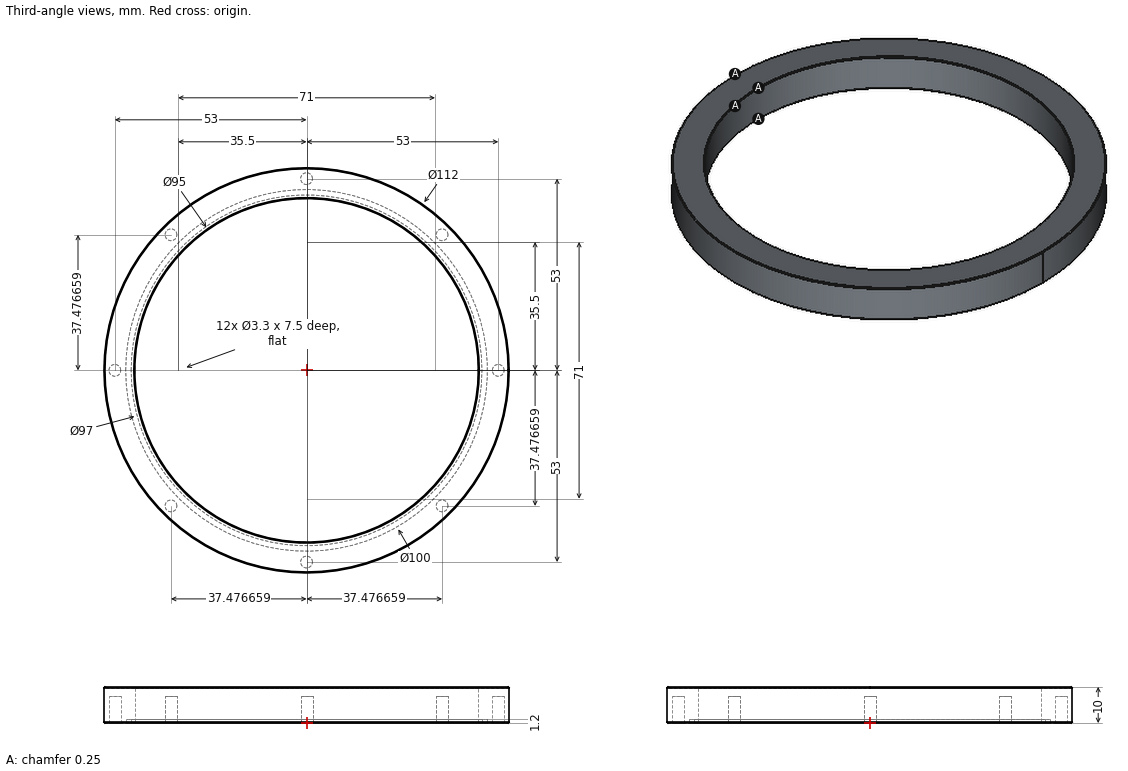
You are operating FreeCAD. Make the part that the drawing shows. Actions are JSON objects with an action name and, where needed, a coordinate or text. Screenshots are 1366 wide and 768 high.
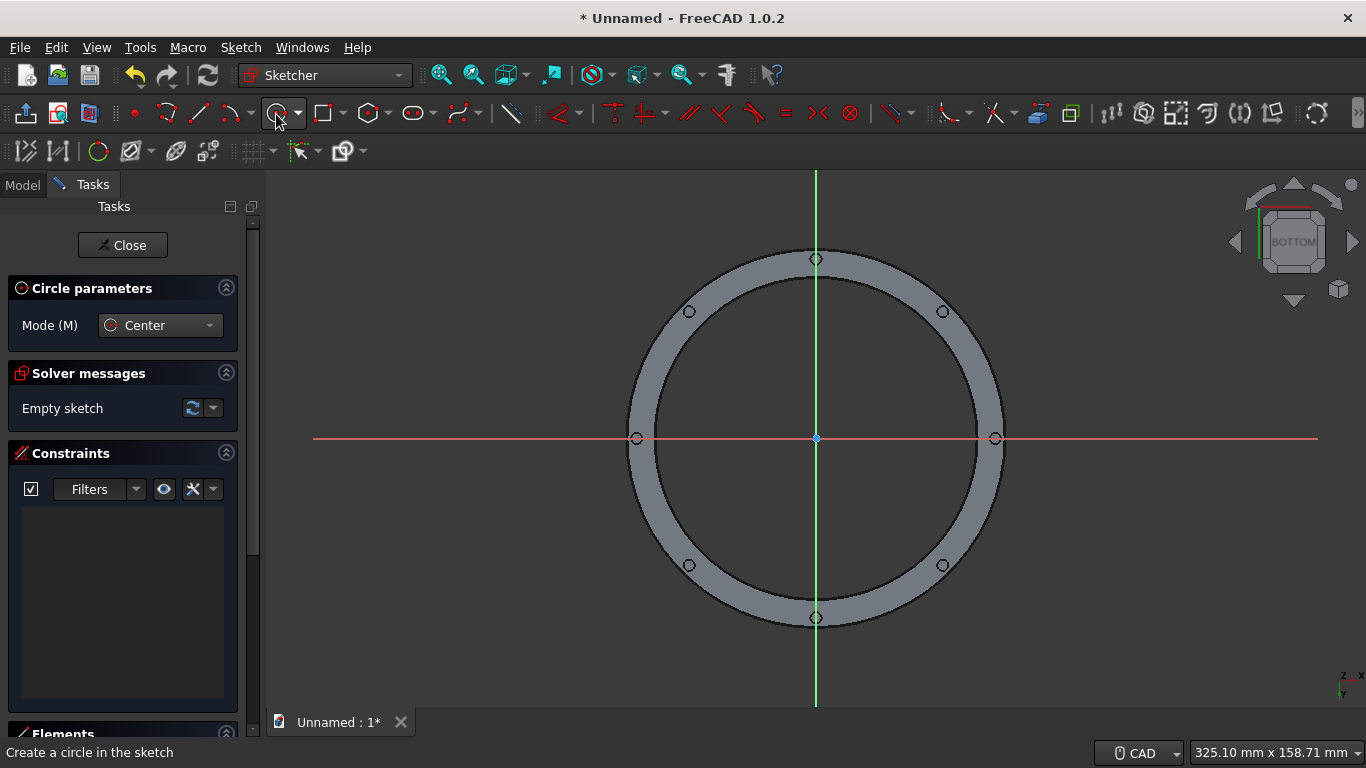
{"action": "left_click", "coordinate": [816, 438]}
{"action": "mouse_move", "coordinate": [936, 319]}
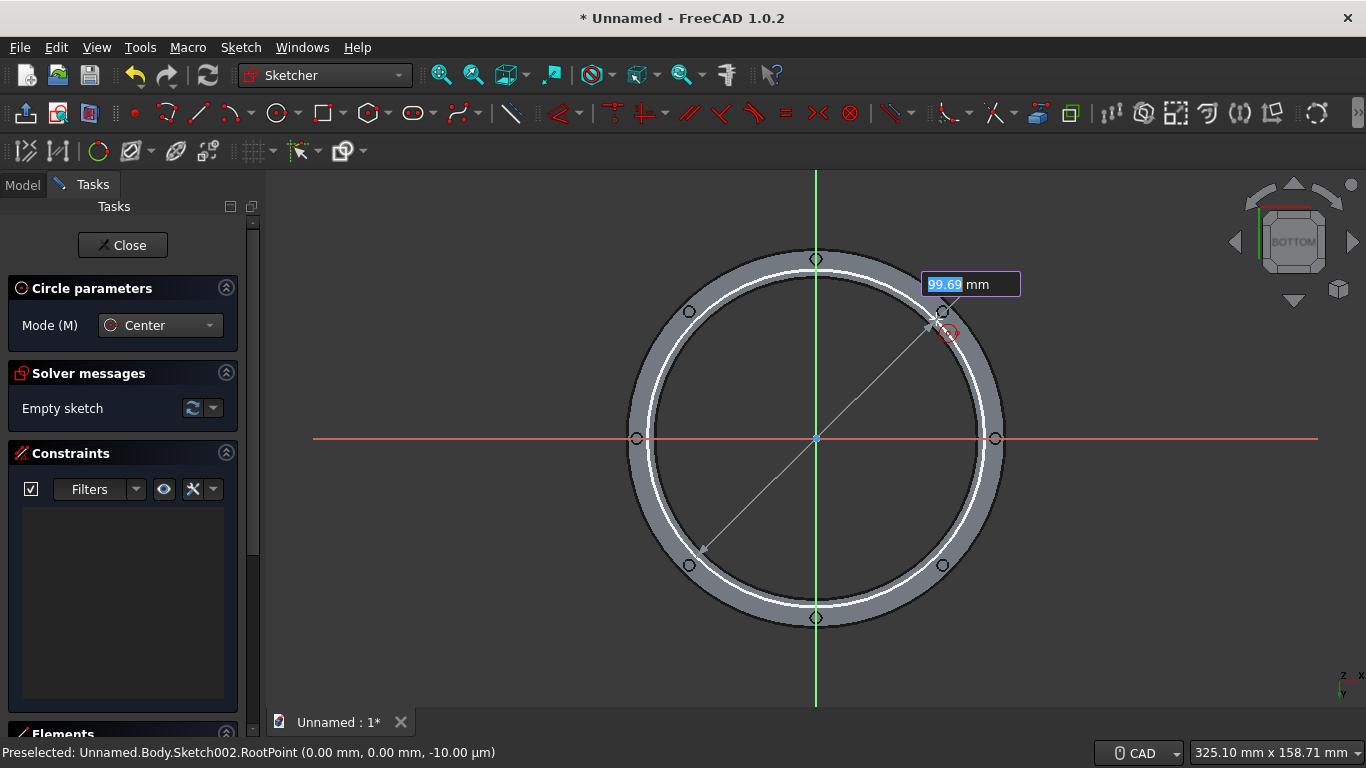
{"action": "type", "text": "100"}
{"action": "key", "text": "Return"}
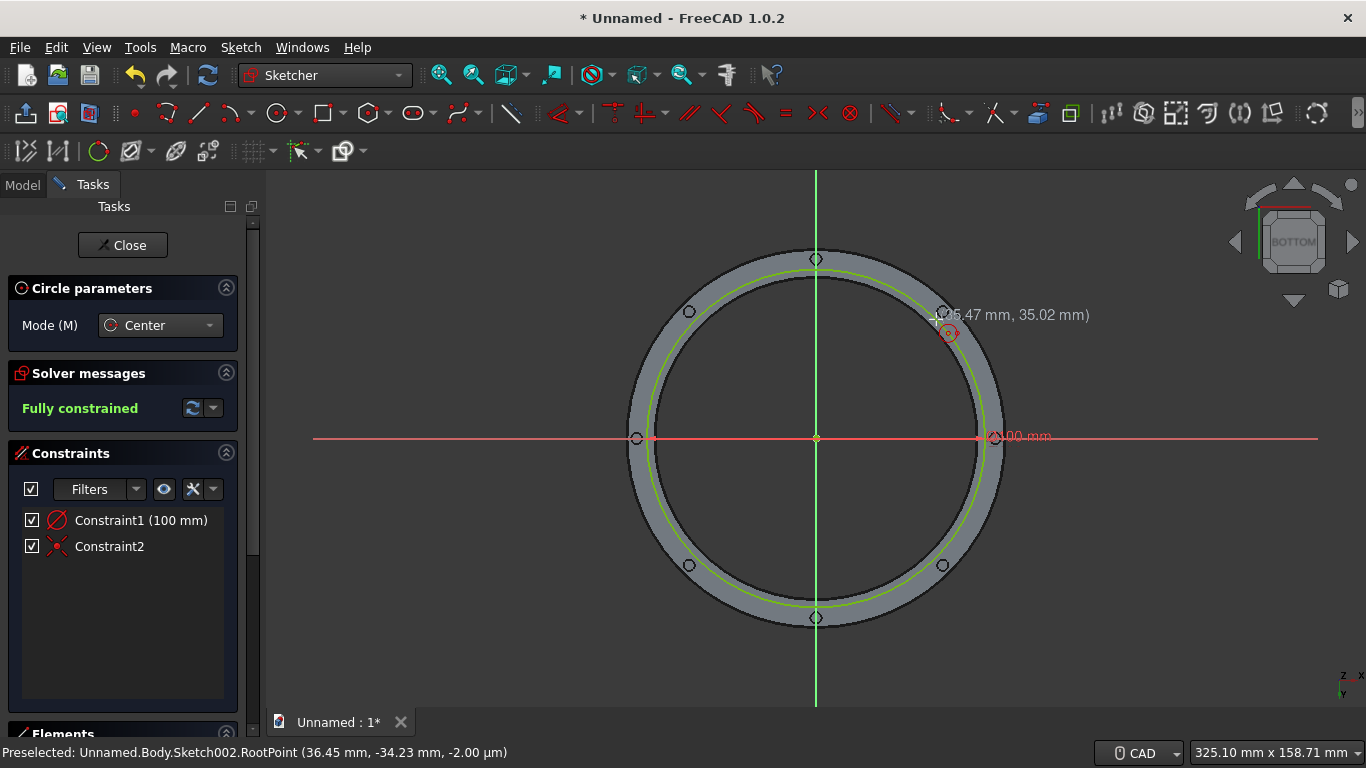
{"action": "left_click", "coordinate": [816, 438]}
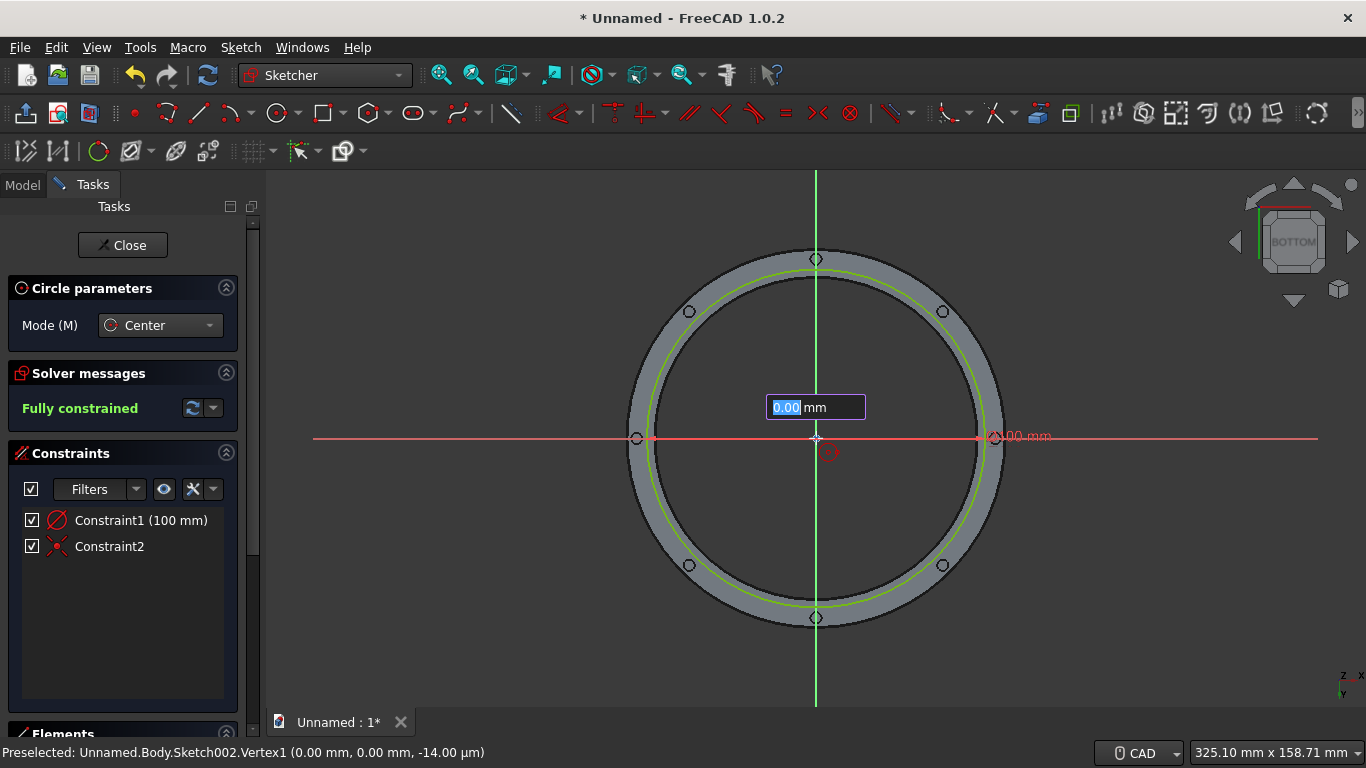
{"action": "scroll", "coordinate": [872, 284], "scroll_direction": "up", "scroll_amount": 6}
{"action": "mouse_move", "coordinate": [871, 284]}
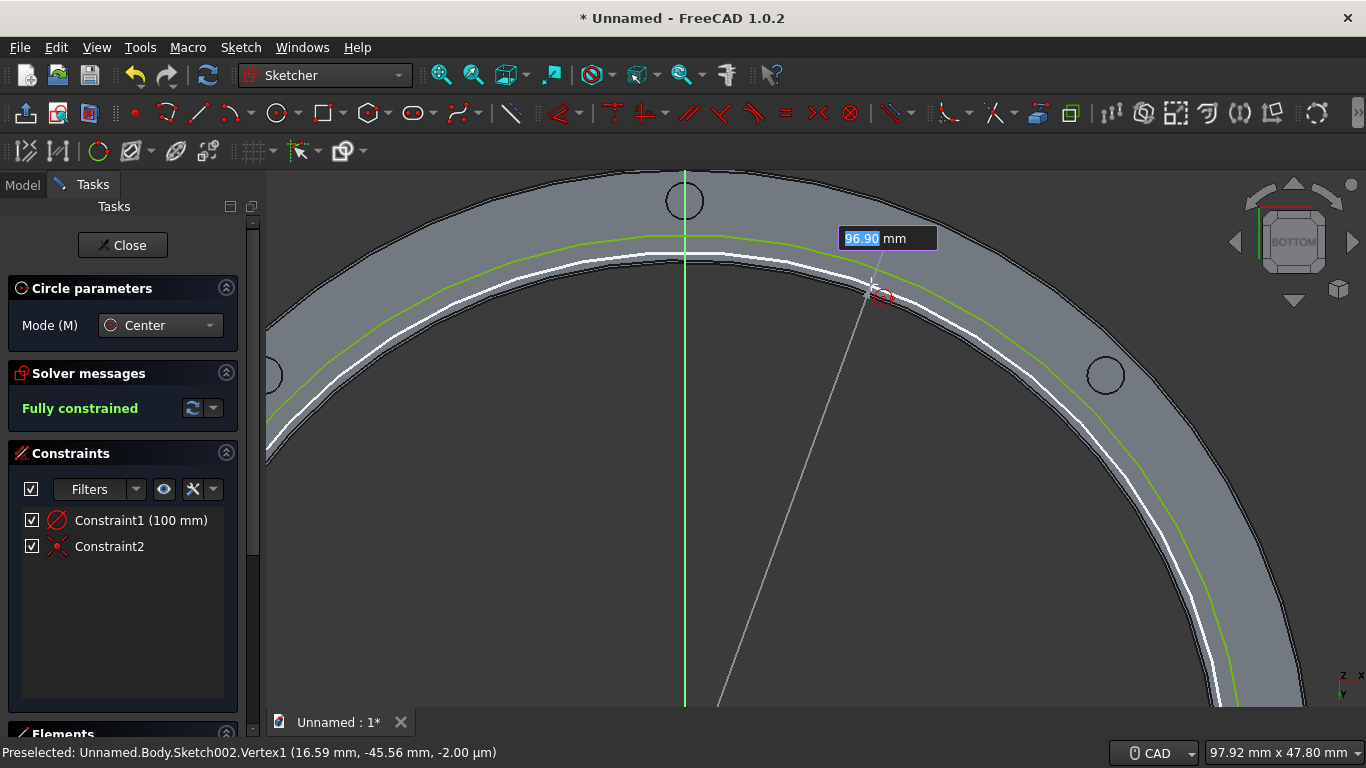
{"action": "type", "text": "97"}
{"action": "key", "text": "Return"}
{"action": "key", "text": "Escape"}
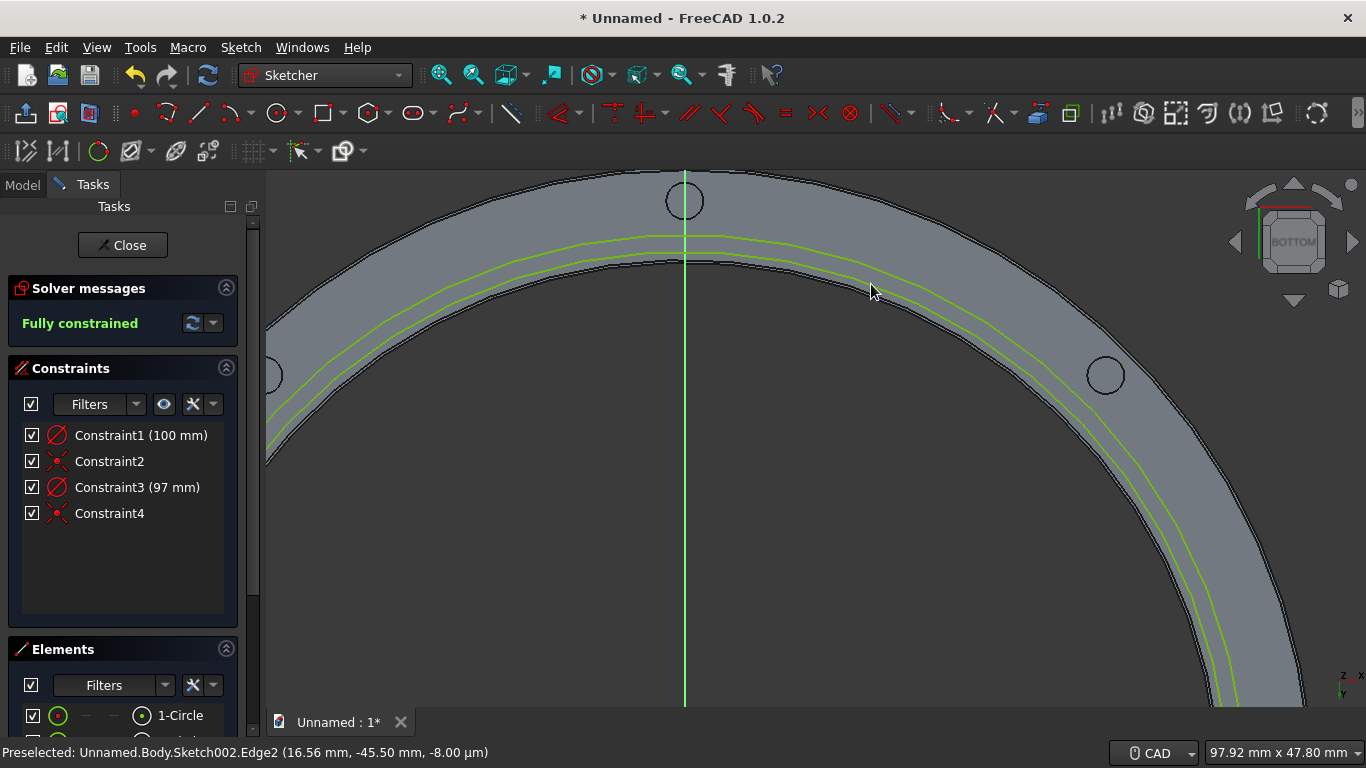
{"action": "left_click", "coordinate": [123, 245]}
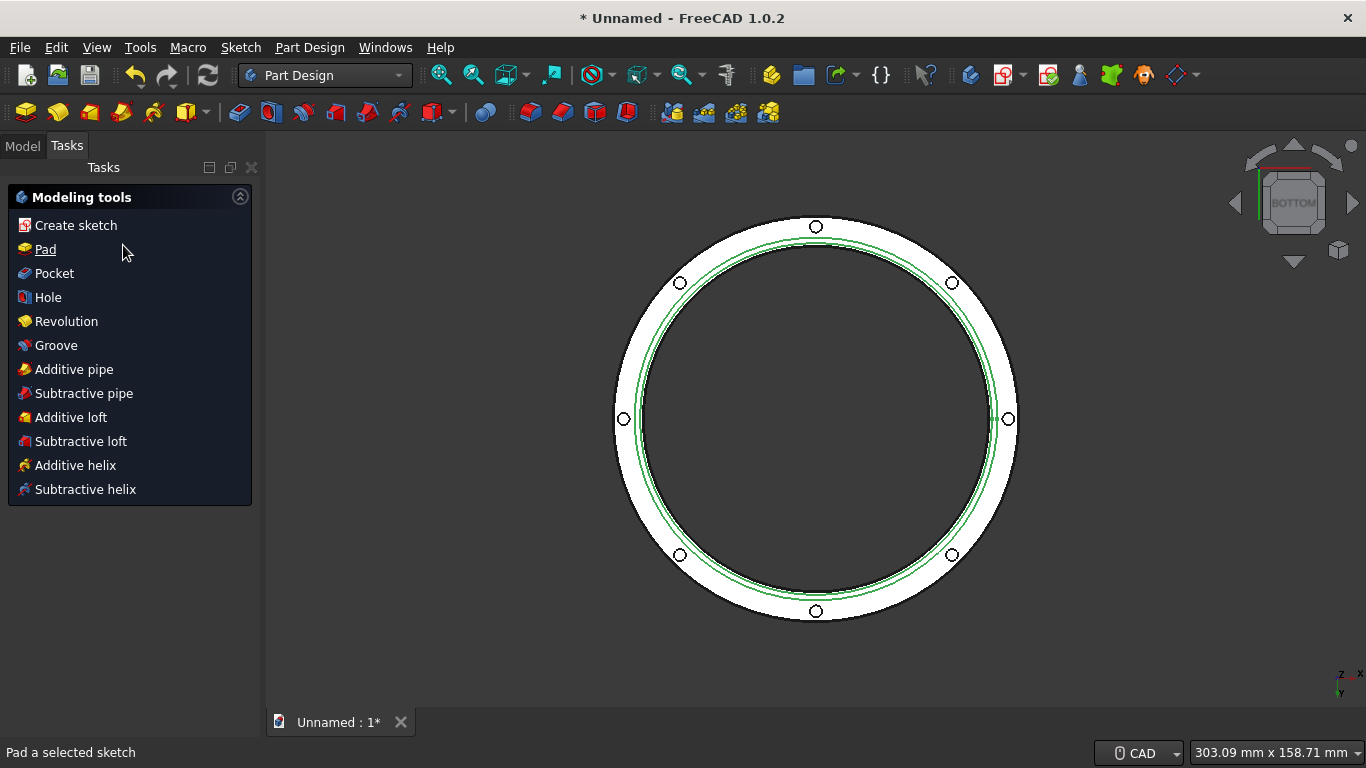
{"action": "left_click", "coordinate": [240, 112]}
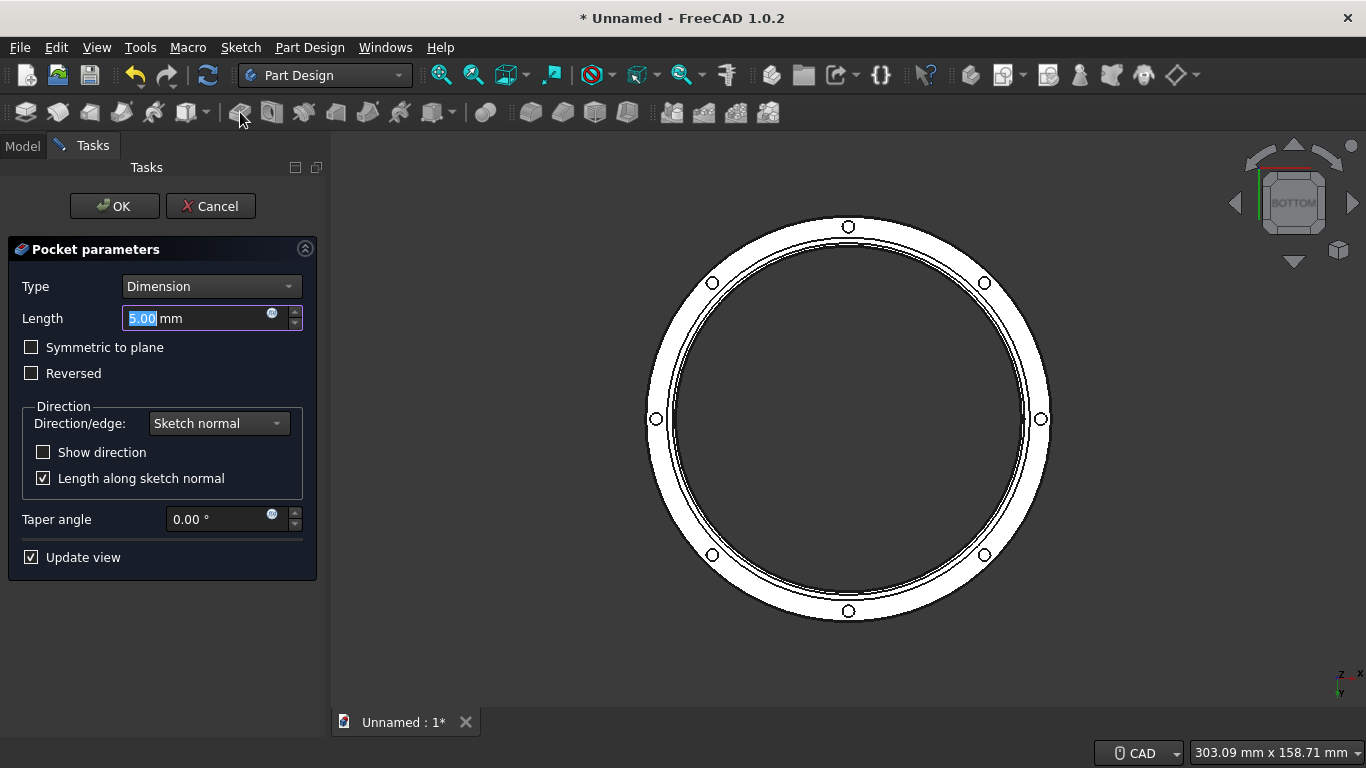
{"action": "type", "text": "1.2"}
{"action": "key", "text": "Tab"}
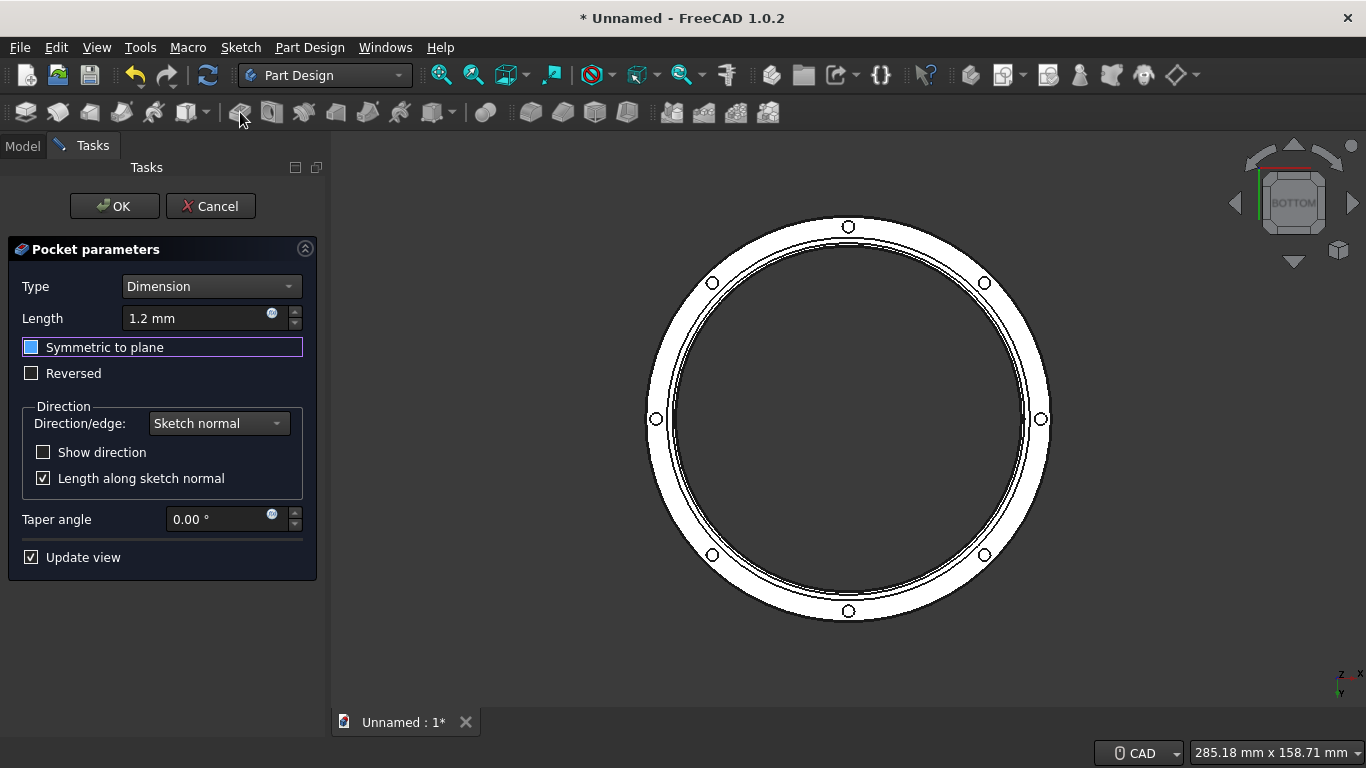
{"action": "left_click", "coordinate": [115, 206]}